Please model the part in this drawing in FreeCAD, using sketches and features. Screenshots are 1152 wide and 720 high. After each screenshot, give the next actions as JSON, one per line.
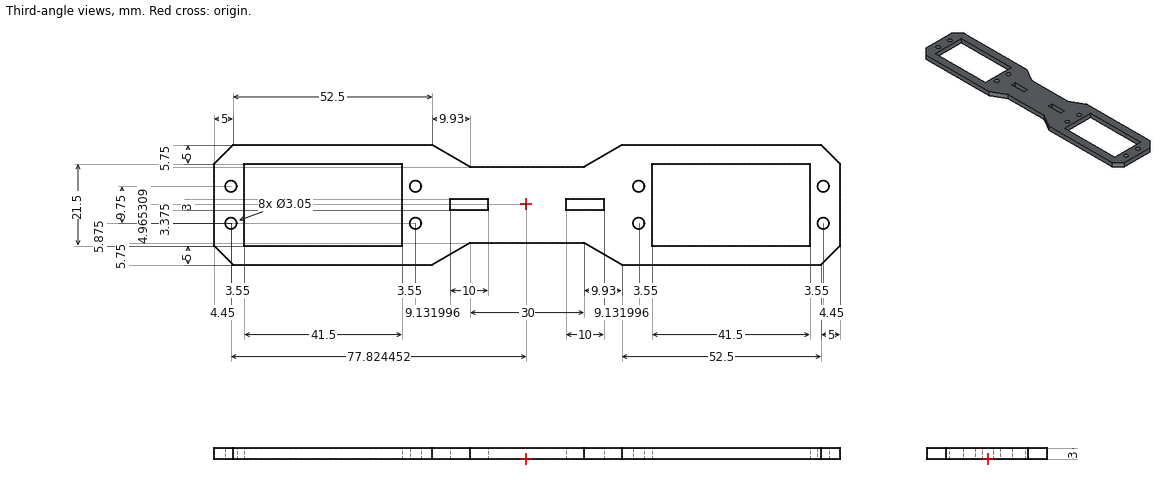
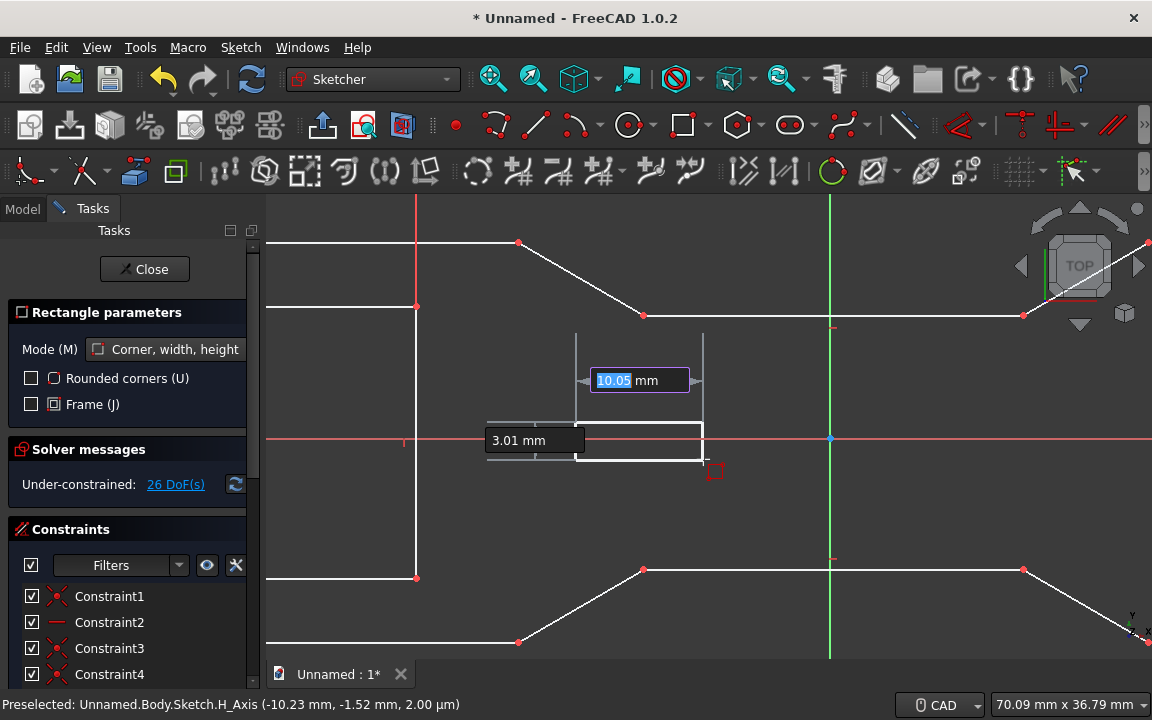
{"action": "type", "text": "10"}
{"action": "key", "text": "Tab"}
{"action": "type", "text": "3"}
{"action": "key", "text": "Return"}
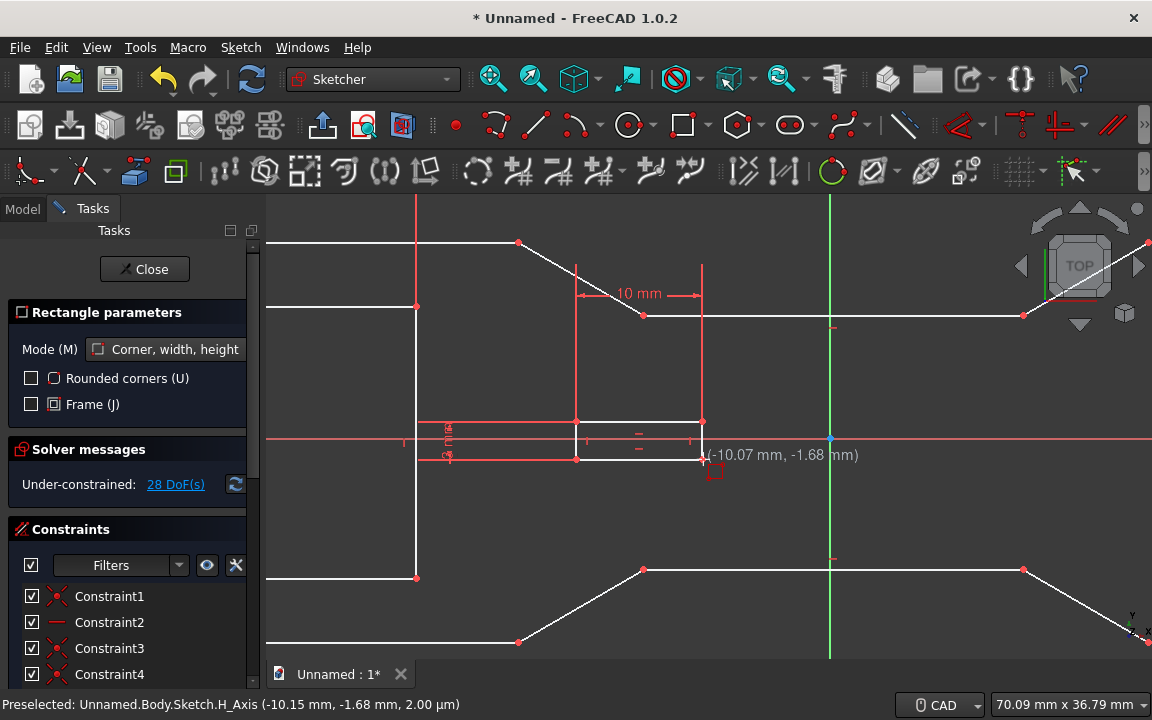
{"action": "left_click", "coordinate": [962, 421]}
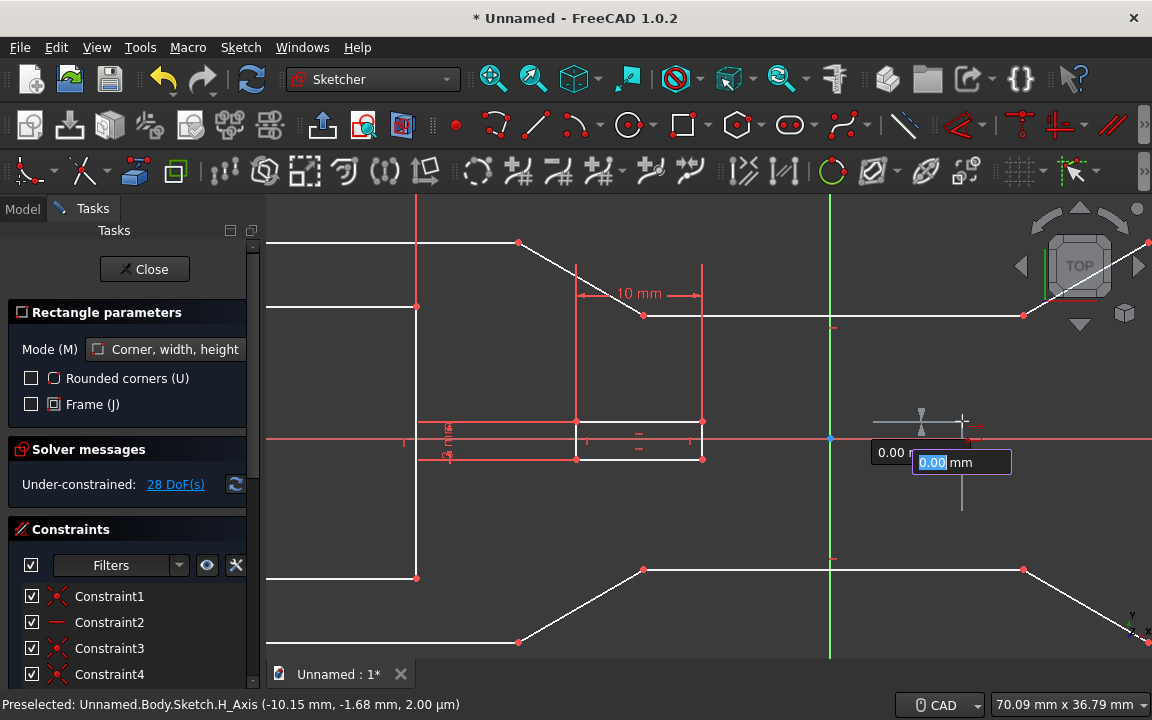
{"action": "scroll", "coordinate": [578, 422], "scroll_direction": "down", "scroll_amount": 7}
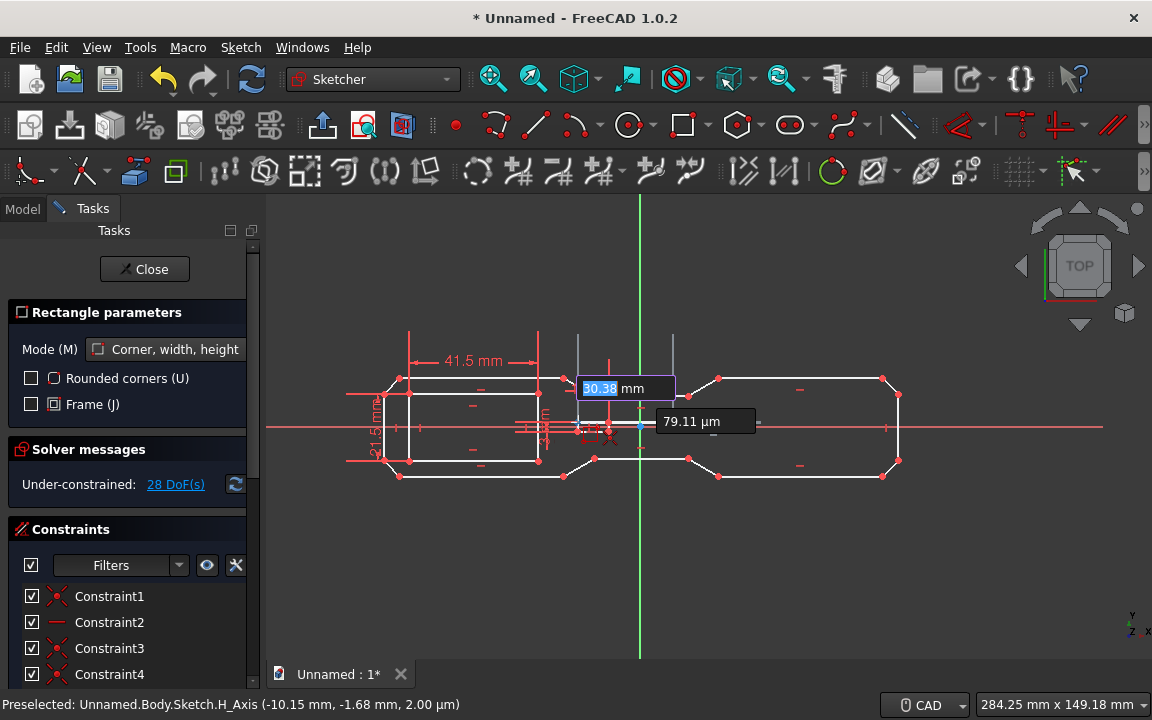
{"action": "scroll", "coordinate": [704, 431], "scroll_direction": "up", "scroll_amount": 6}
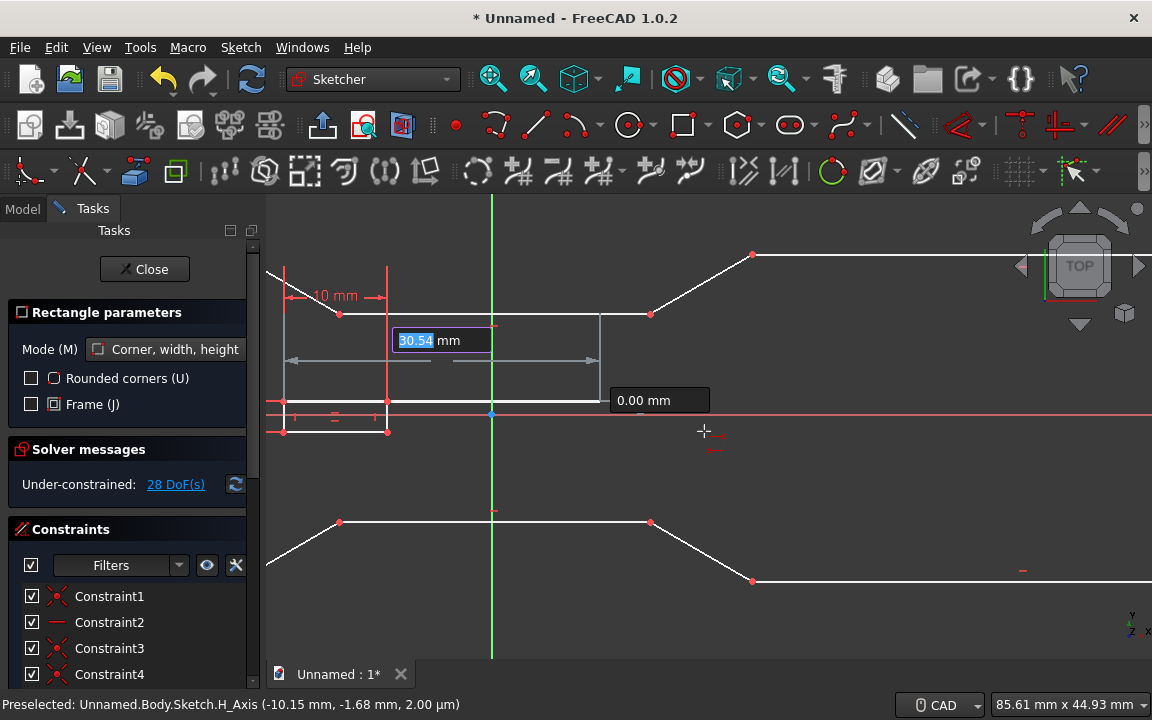
{"action": "left_click", "coordinate": [703, 431]}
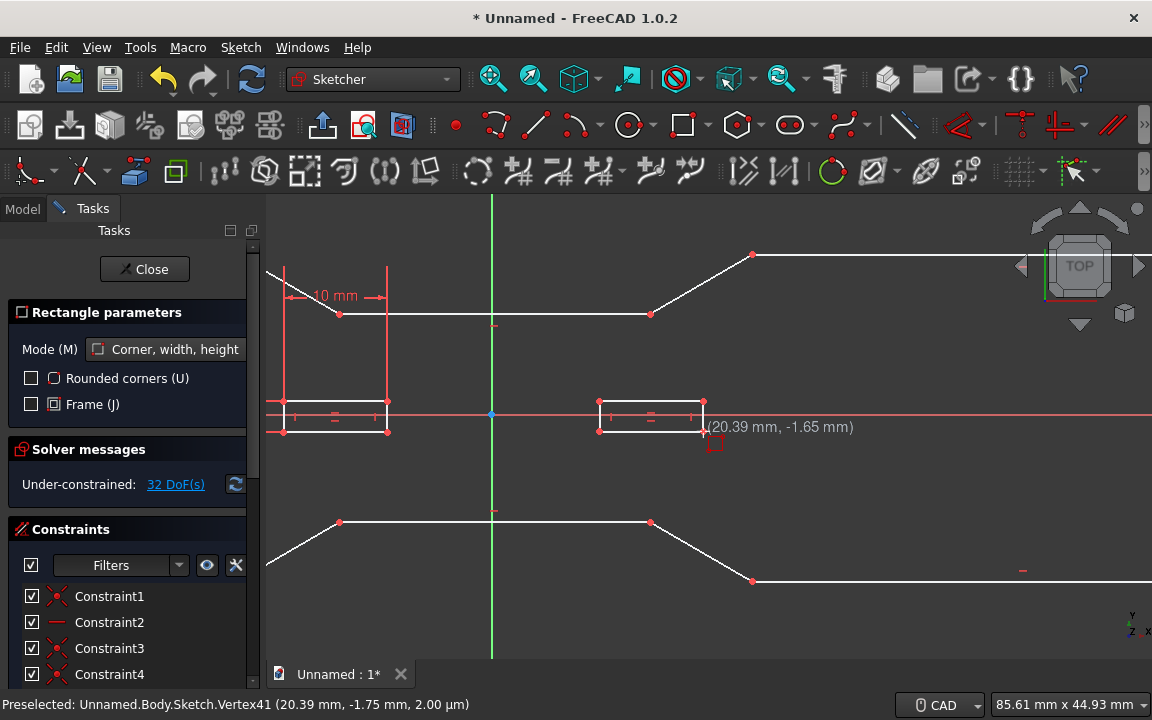
{"action": "left_click", "coordinate": [834, 305]}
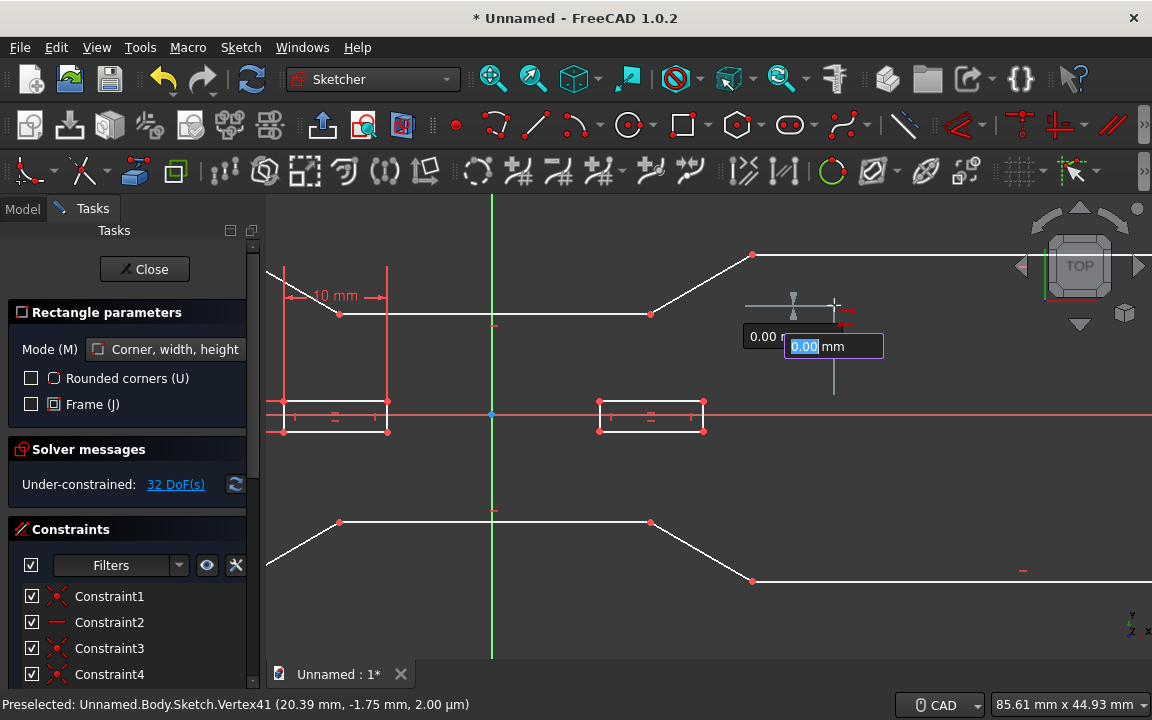
{"action": "scroll", "coordinate": [704, 431], "scroll_direction": "down", "scroll_amount": 6}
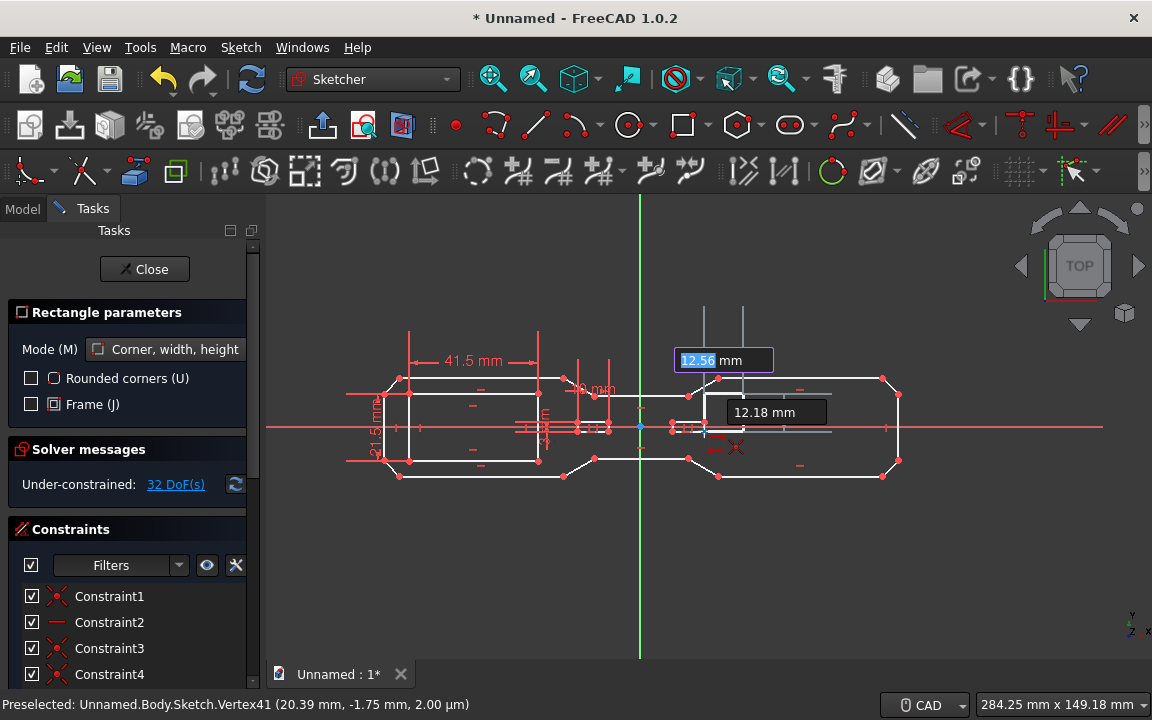
{"action": "left_click", "coordinate": [873, 460]}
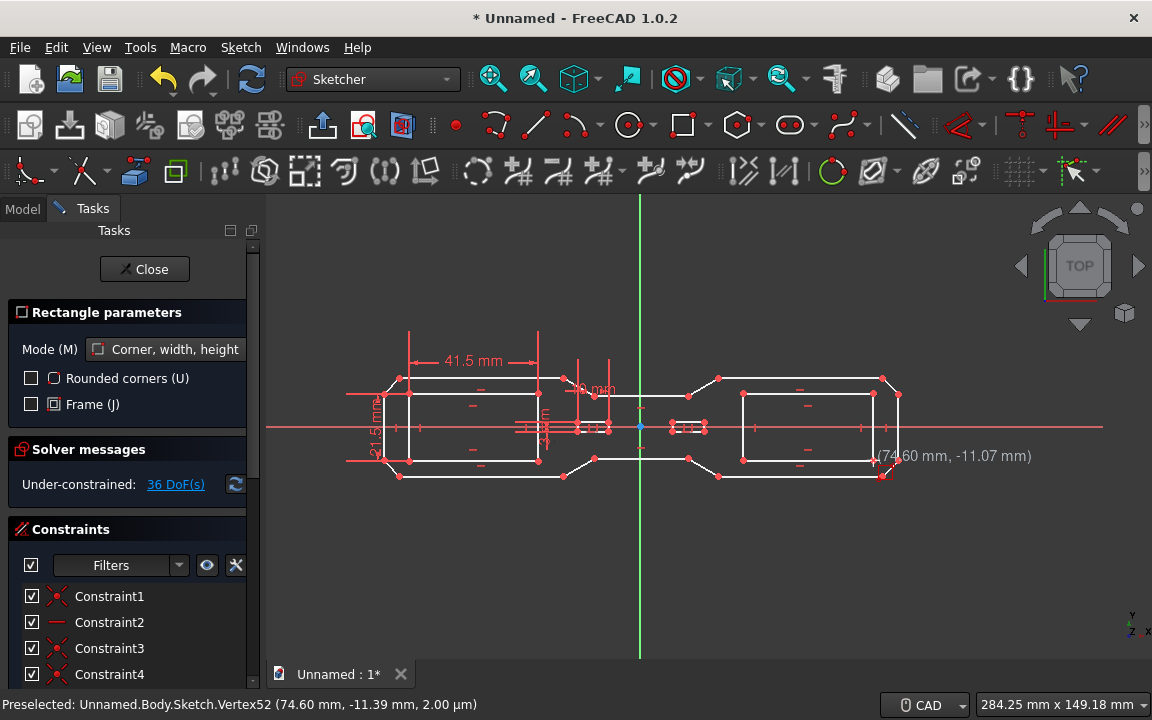
{"action": "left_click", "coordinate": [630, 126]}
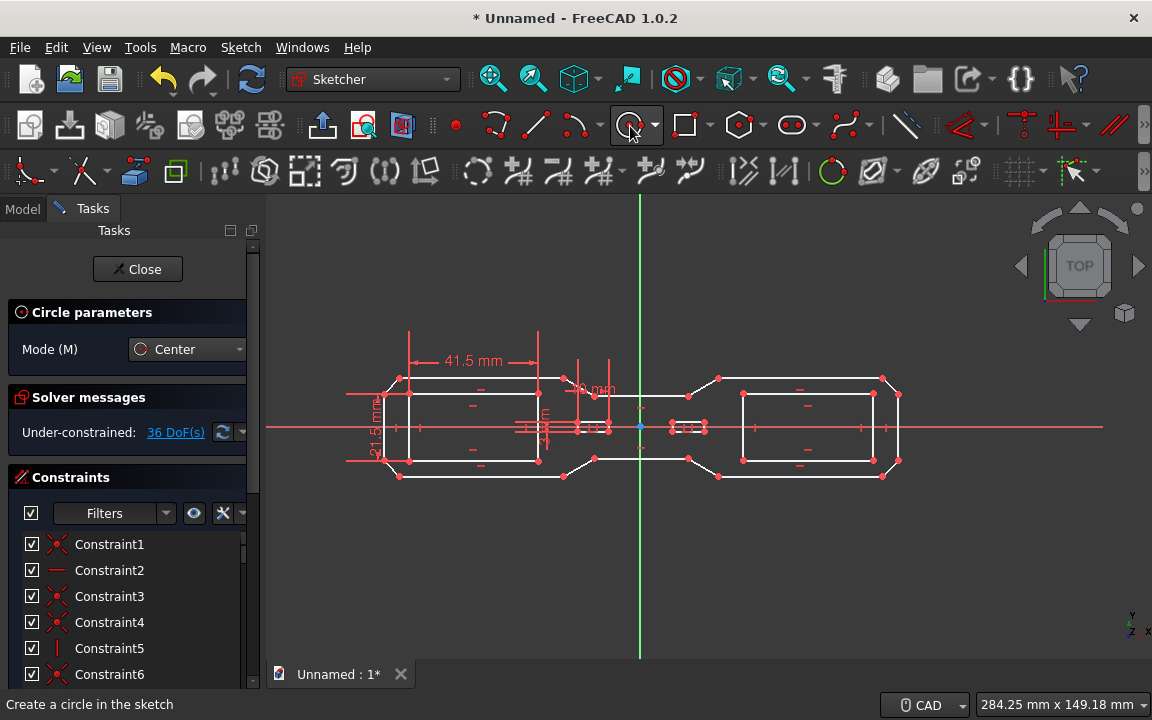
{"action": "scroll", "coordinate": [398, 442], "scroll_direction": "up", "scroll_amount": 8}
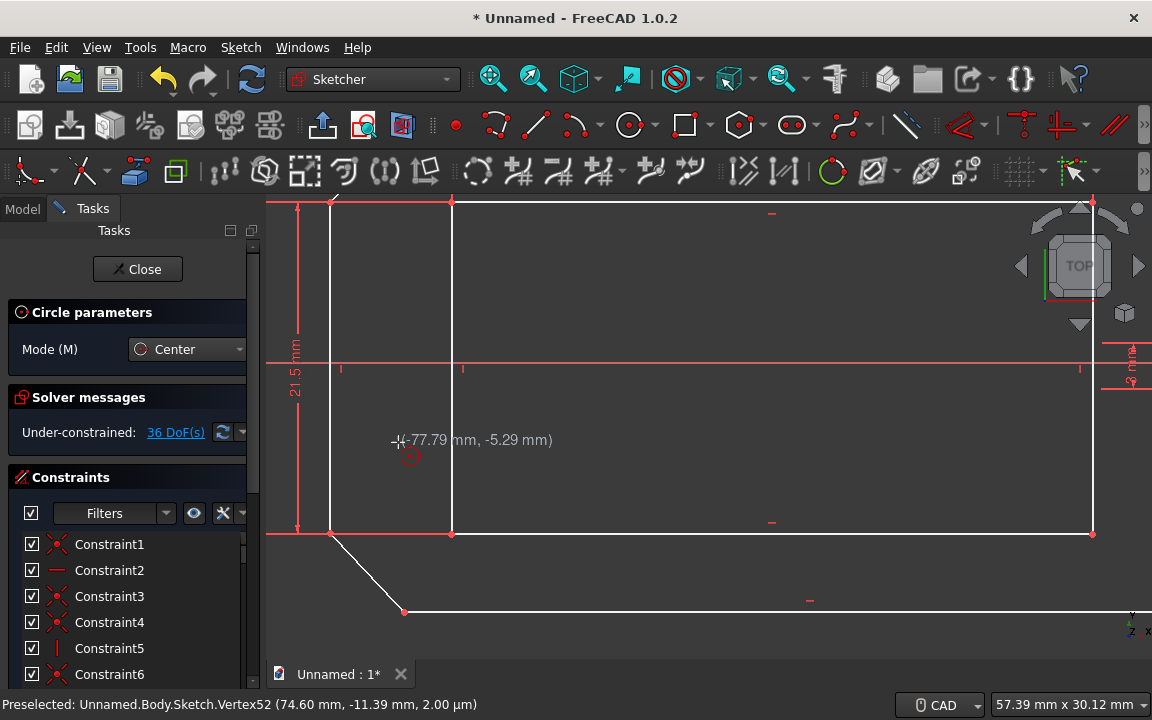
{"action": "scroll", "coordinate": [398, 442], "scroll_direction": "down", "scroll_amount": 8}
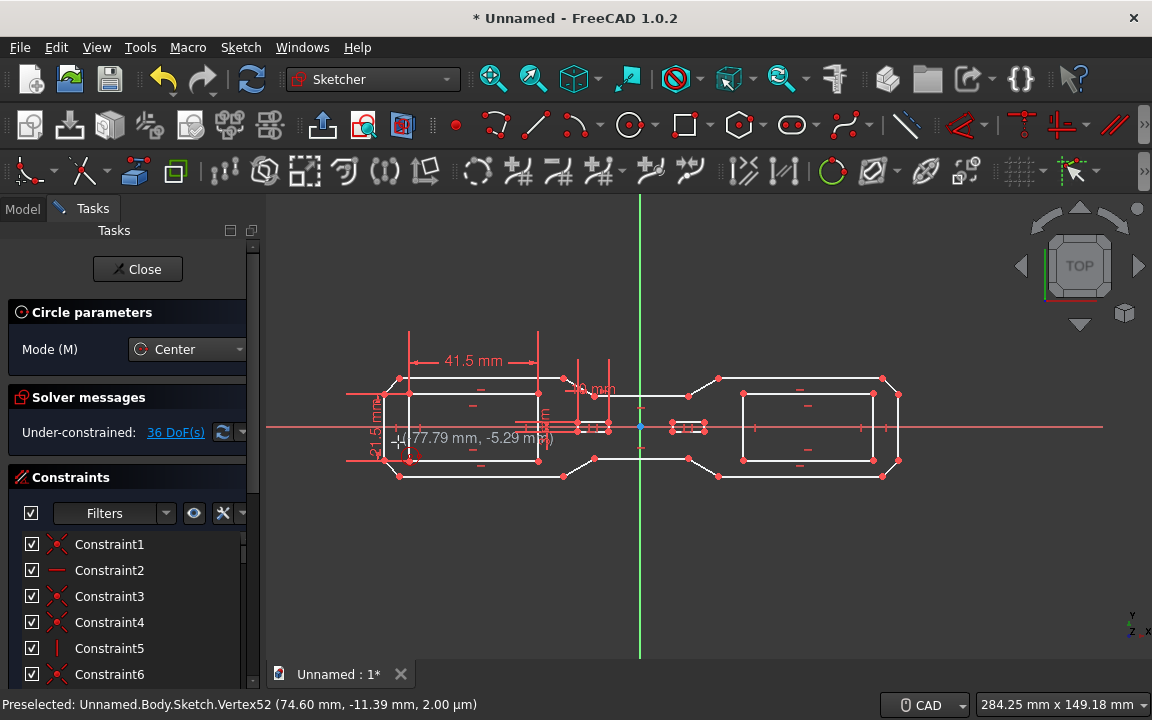
{"action": "scroll", "coordinate": [398, 442], "scroll_direction": "up", "scroll_amount": 2}